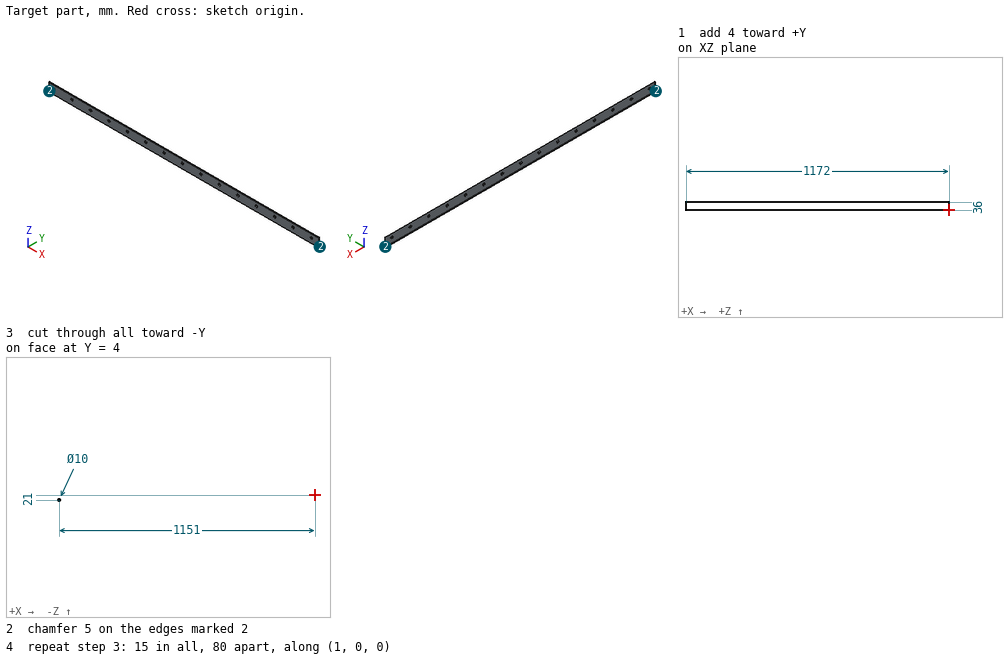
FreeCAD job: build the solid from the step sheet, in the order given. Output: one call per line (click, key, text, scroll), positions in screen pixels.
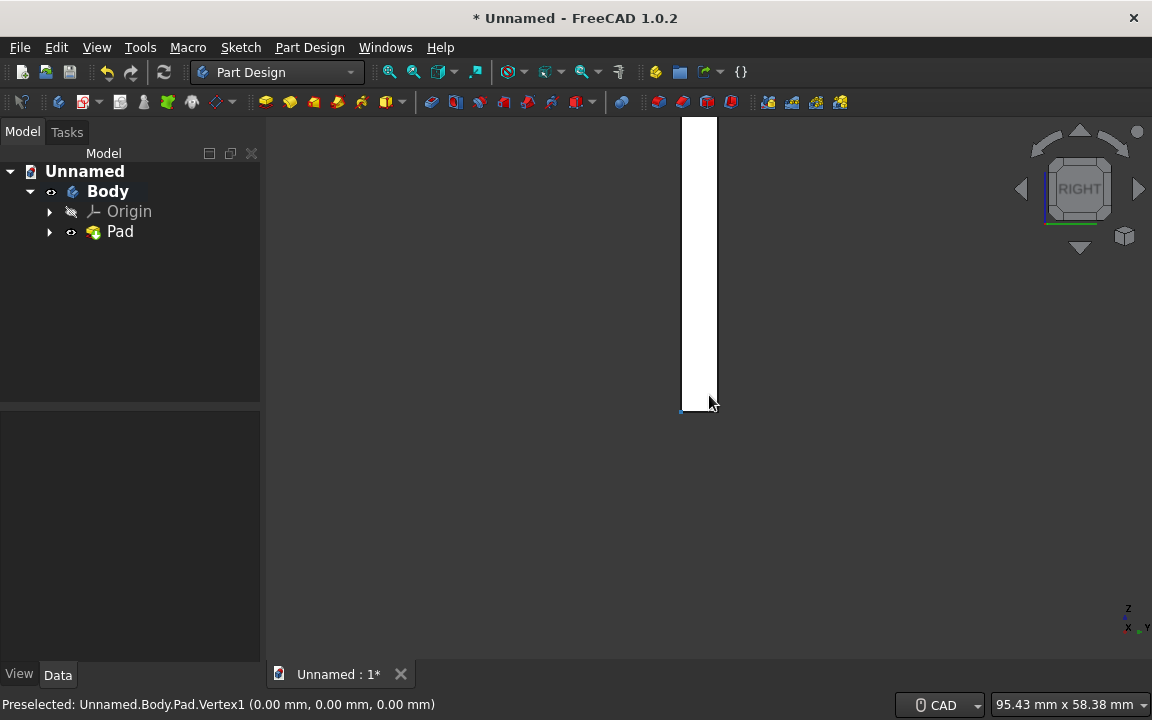
click(699, 411)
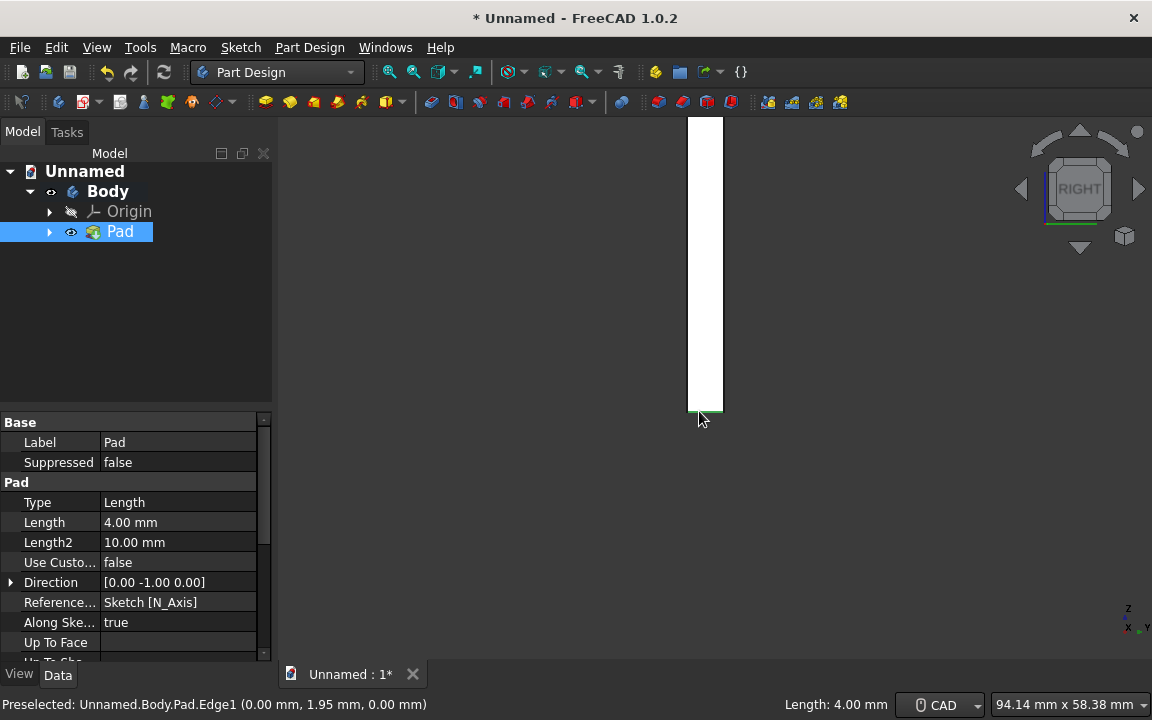
click(390, 72)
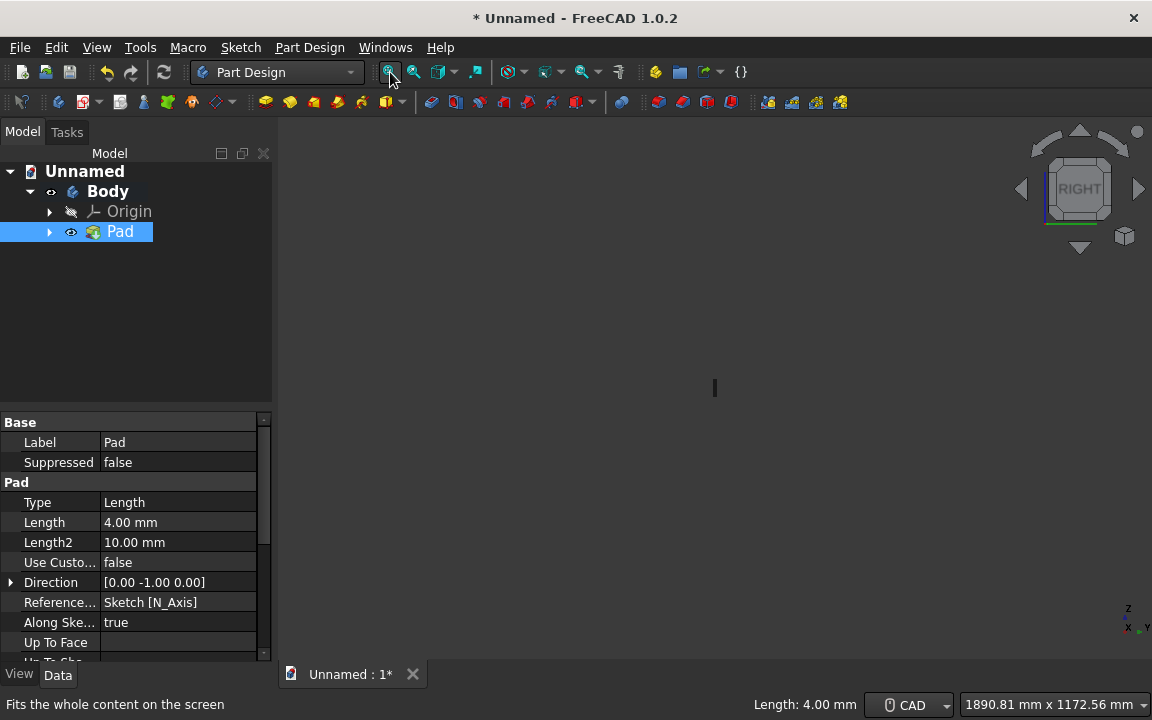
key(5)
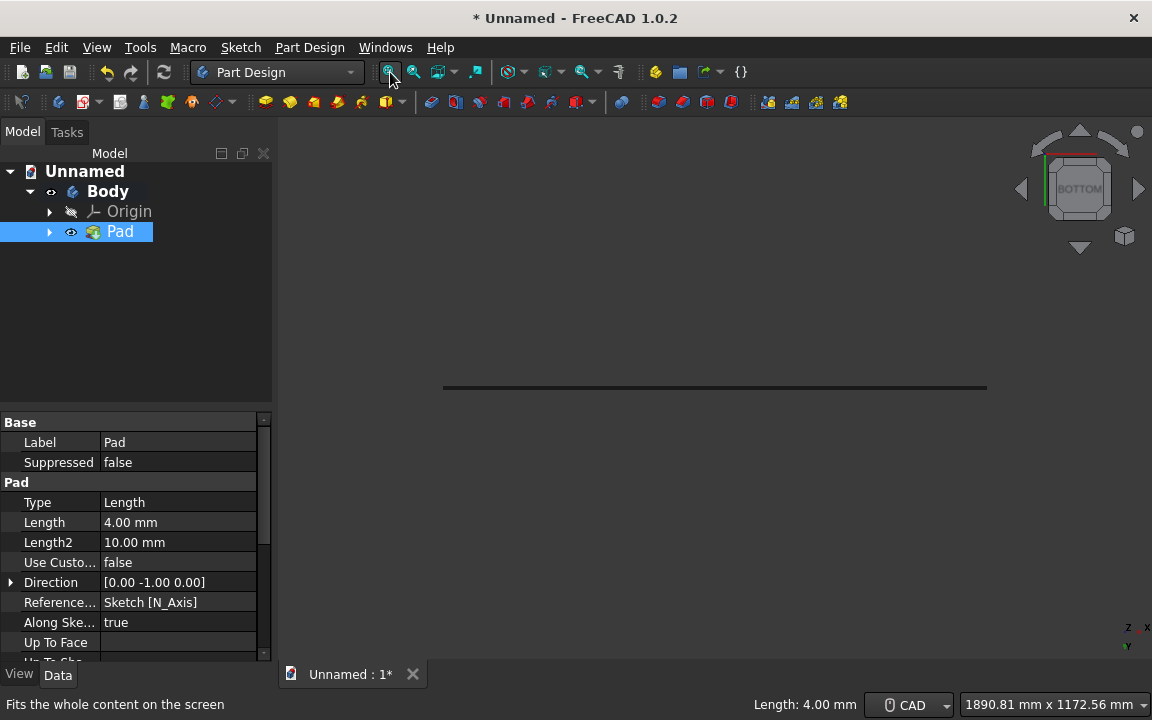
scroll(444, 387, up, 15)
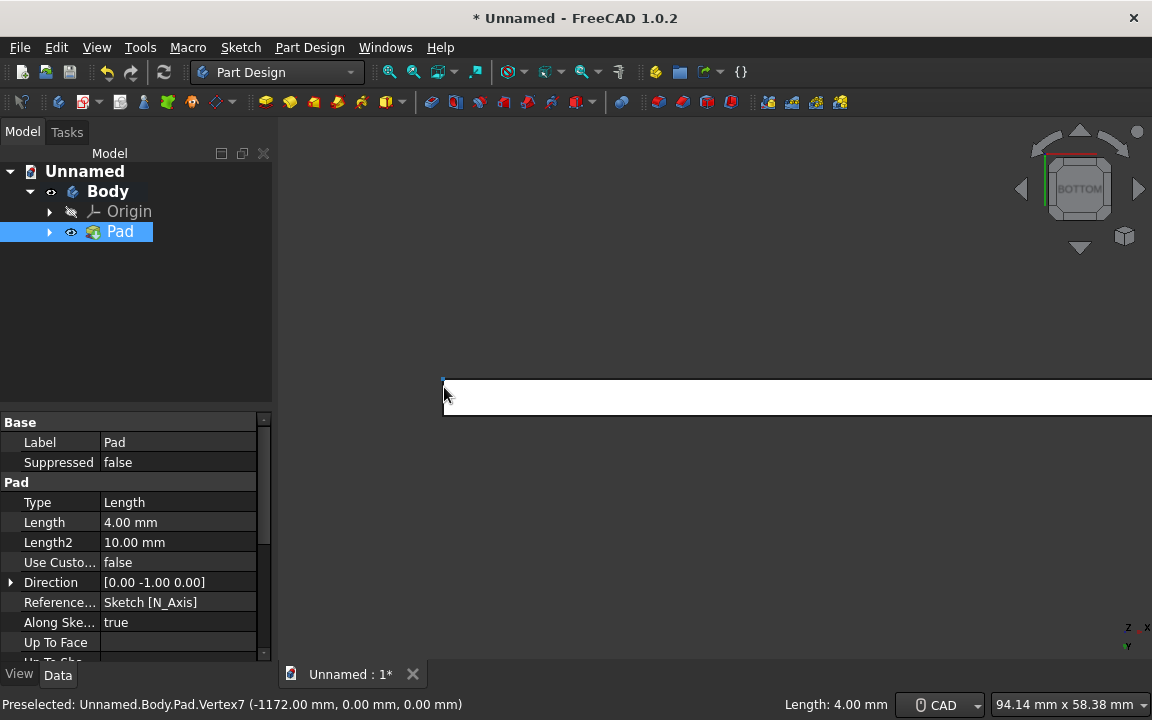
click(443, 397, ctrl)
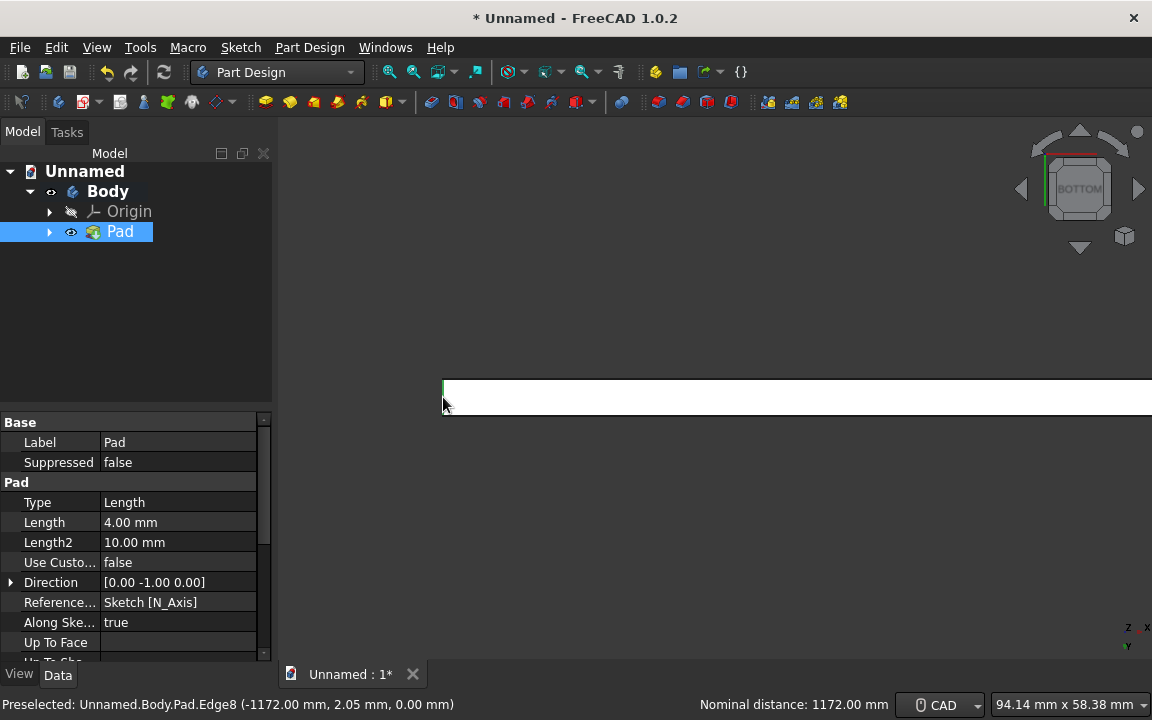
click(684, 102)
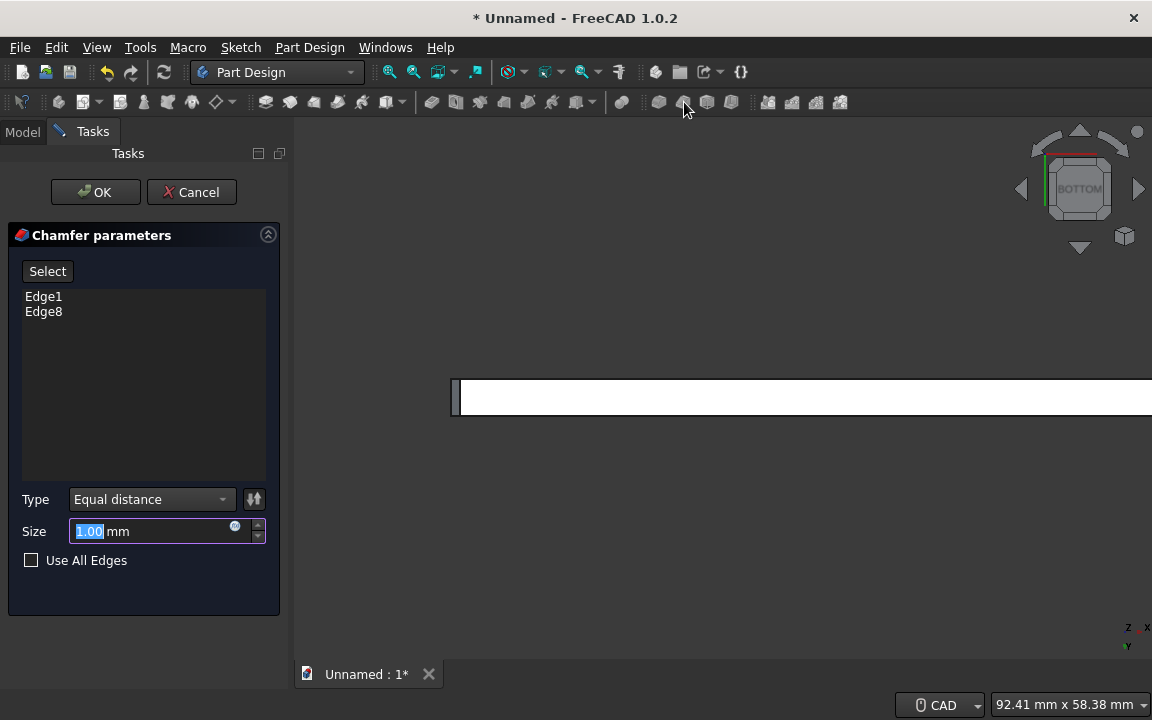
text(5)
key(Tab)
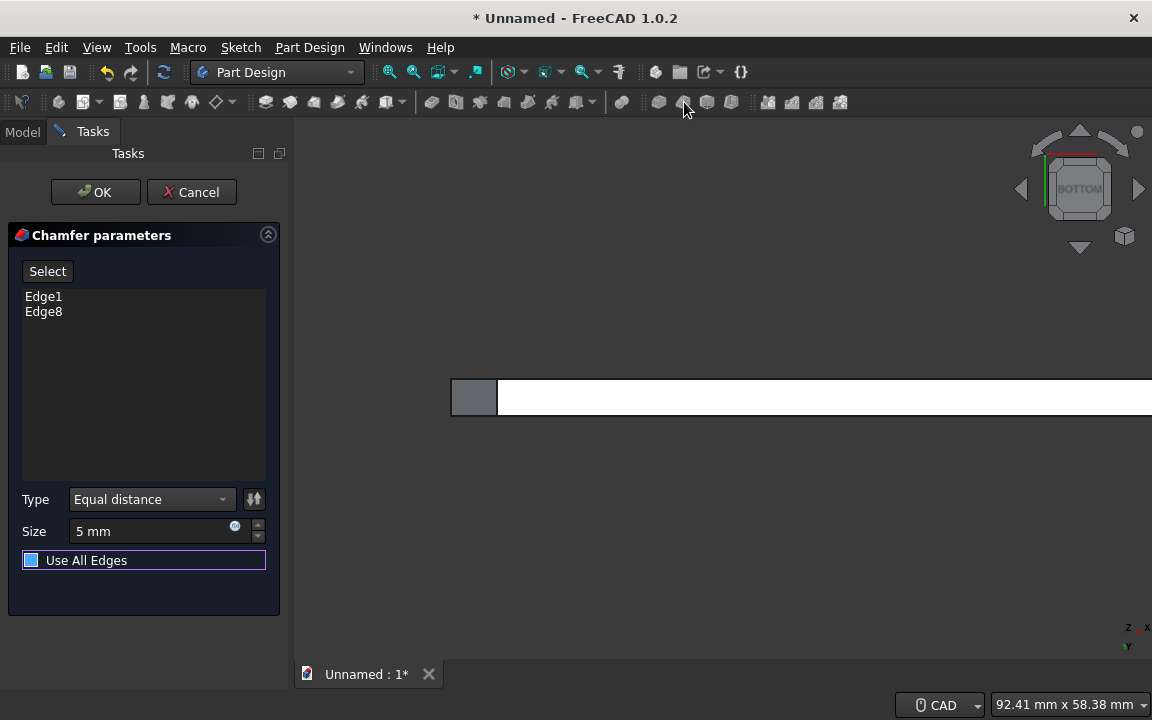
click(96, 192)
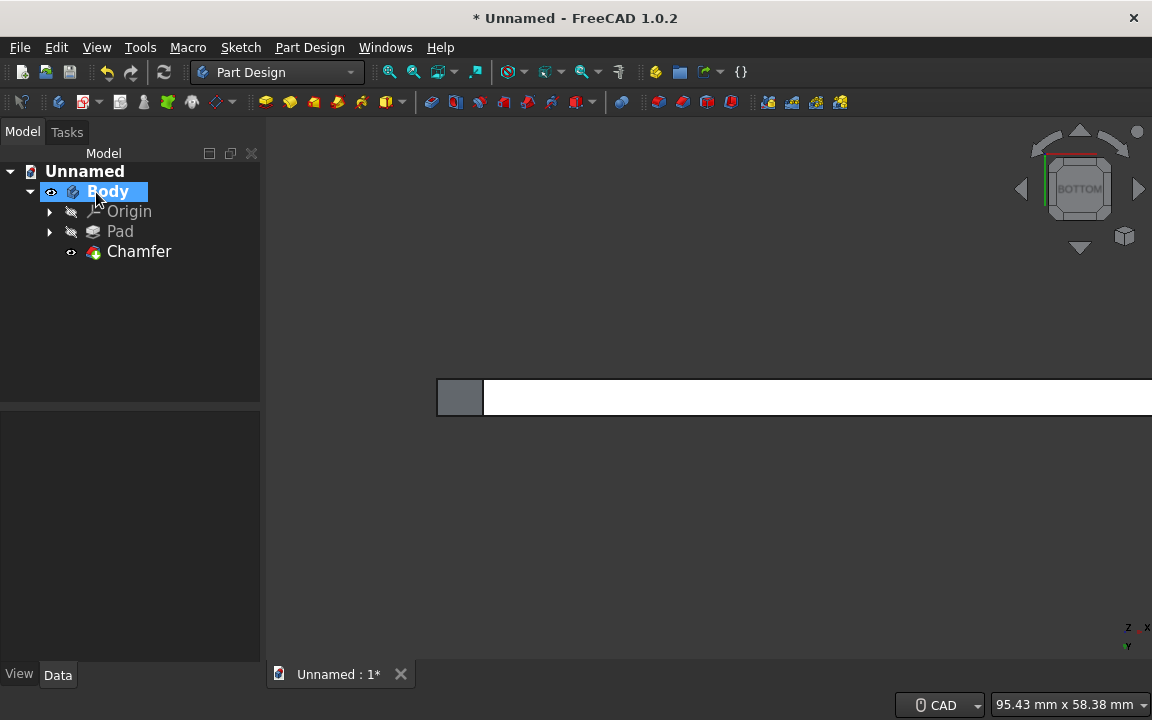
key(v)
key(f)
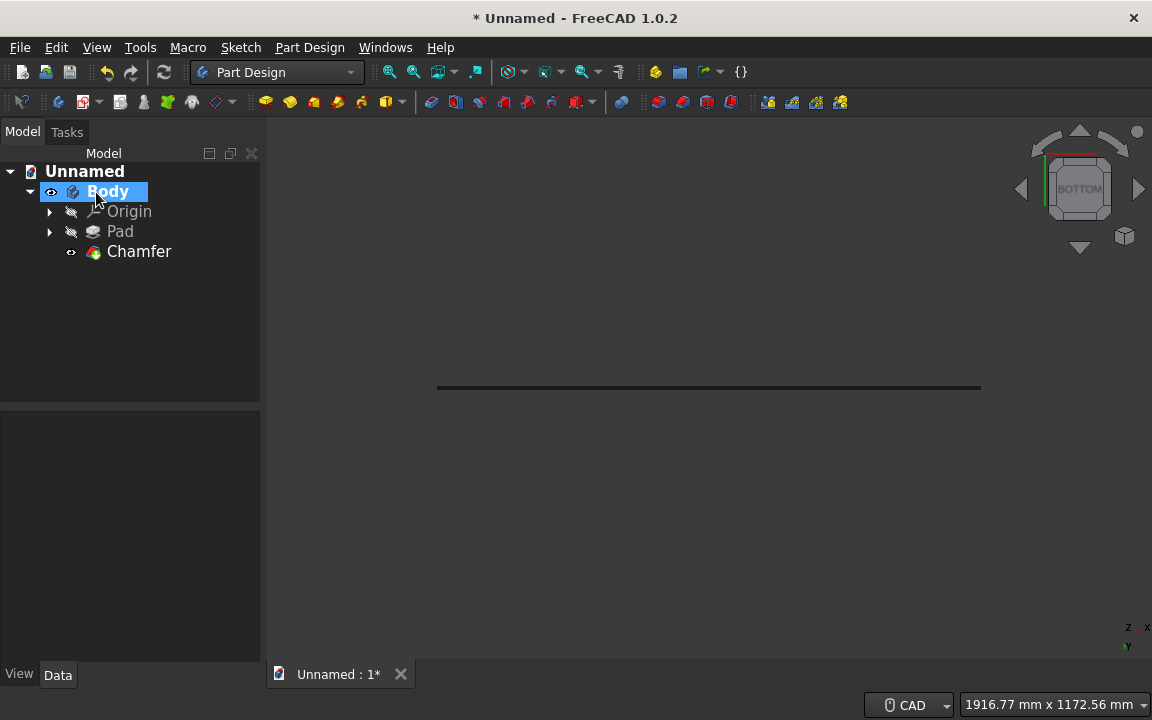
key(4)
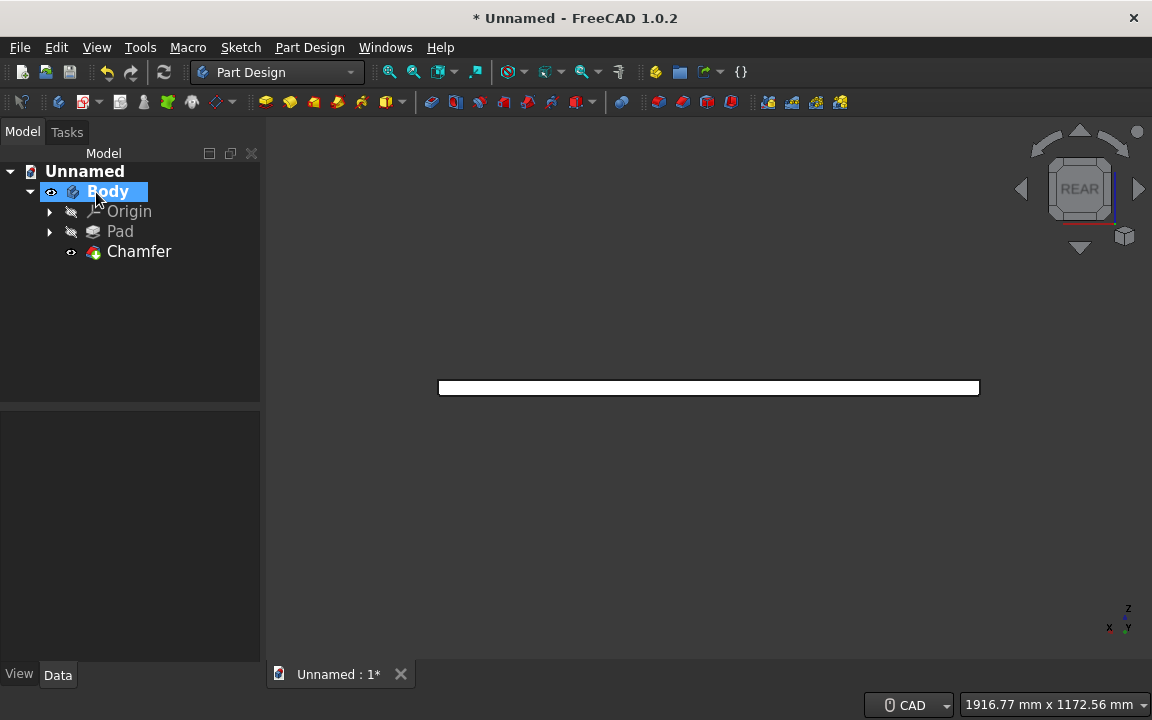
click(477, 387)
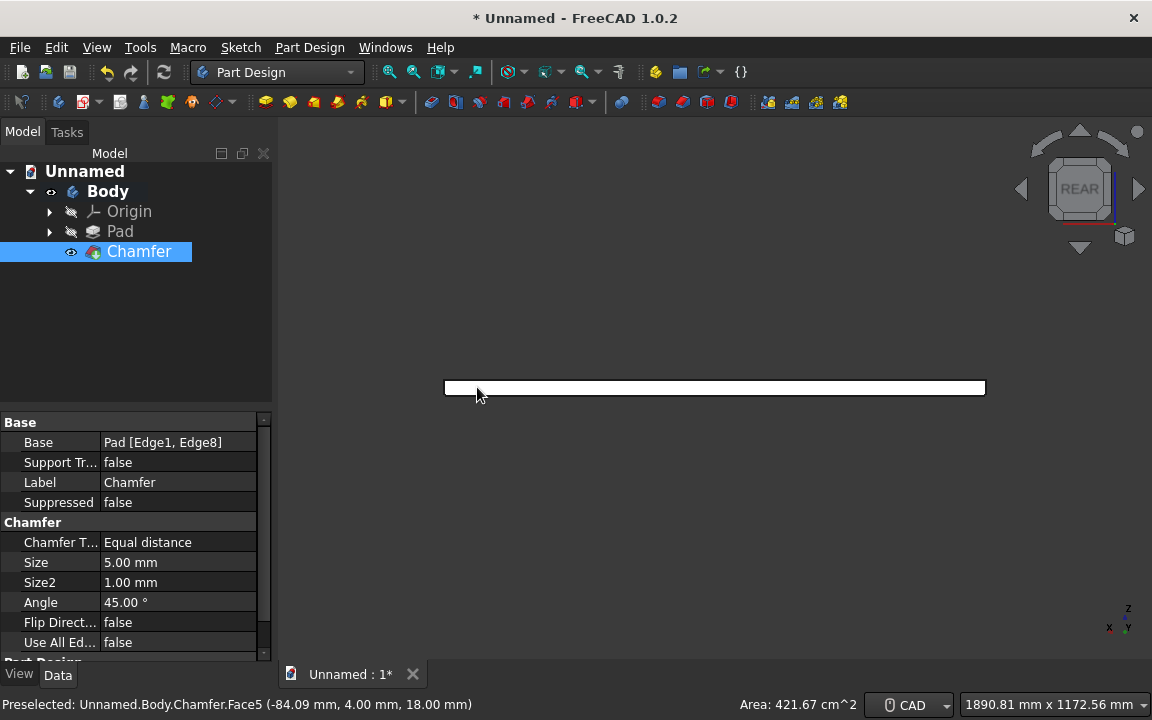
click(84, 102)